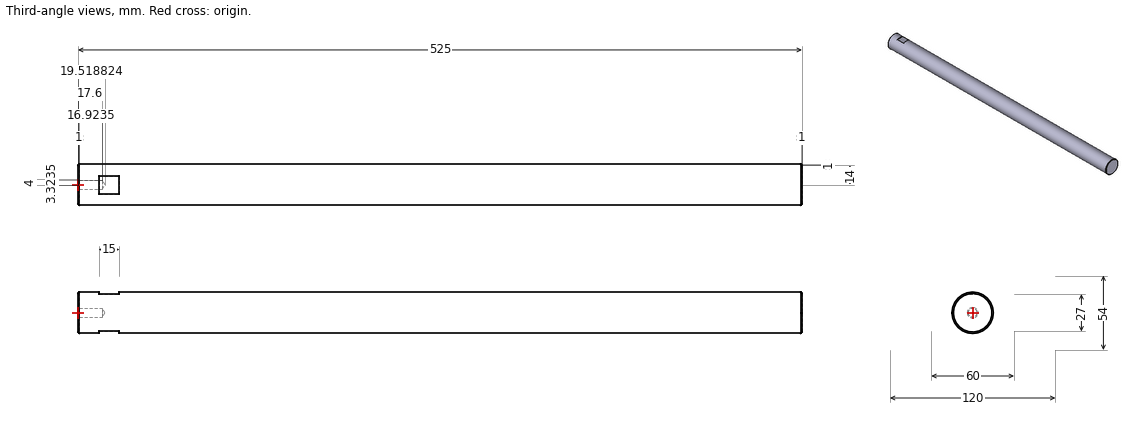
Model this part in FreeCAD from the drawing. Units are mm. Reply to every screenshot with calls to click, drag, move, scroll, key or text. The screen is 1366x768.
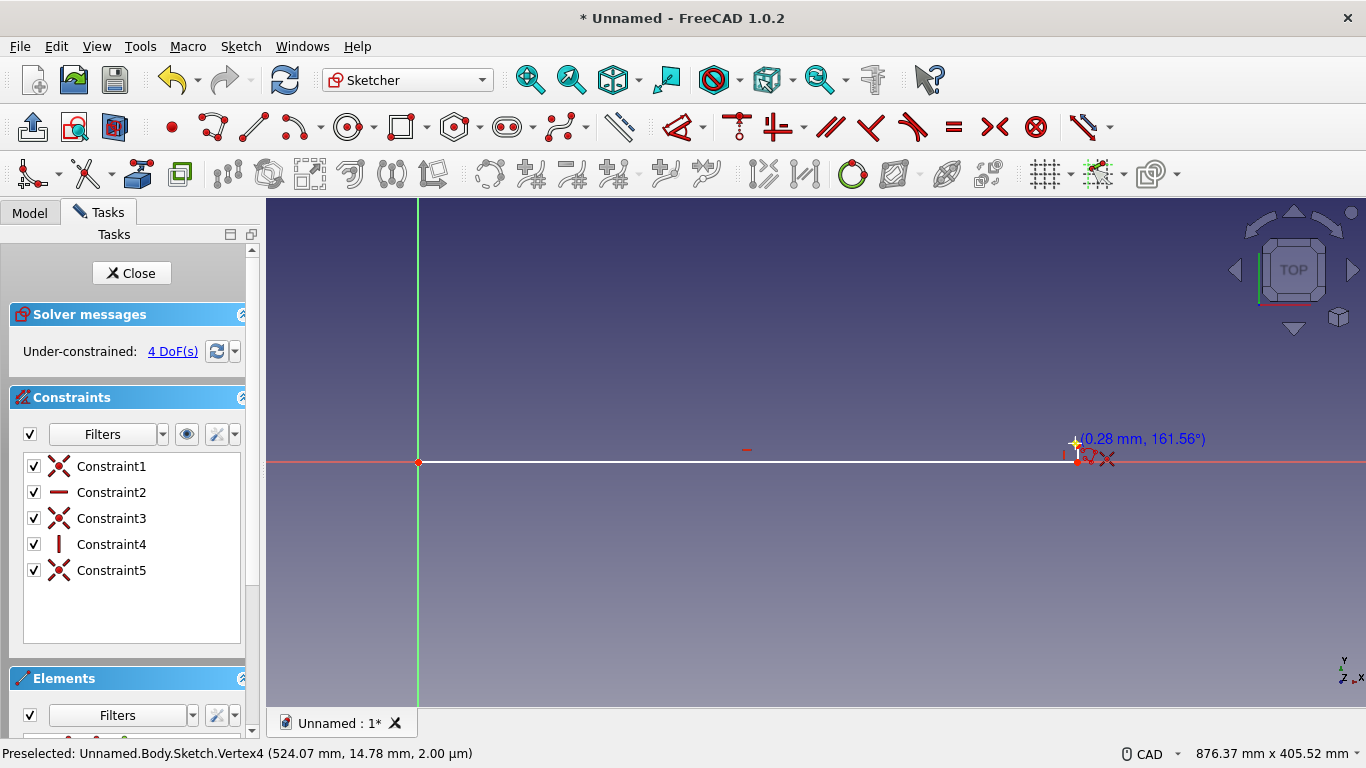
scroll(420, 443, up, 13)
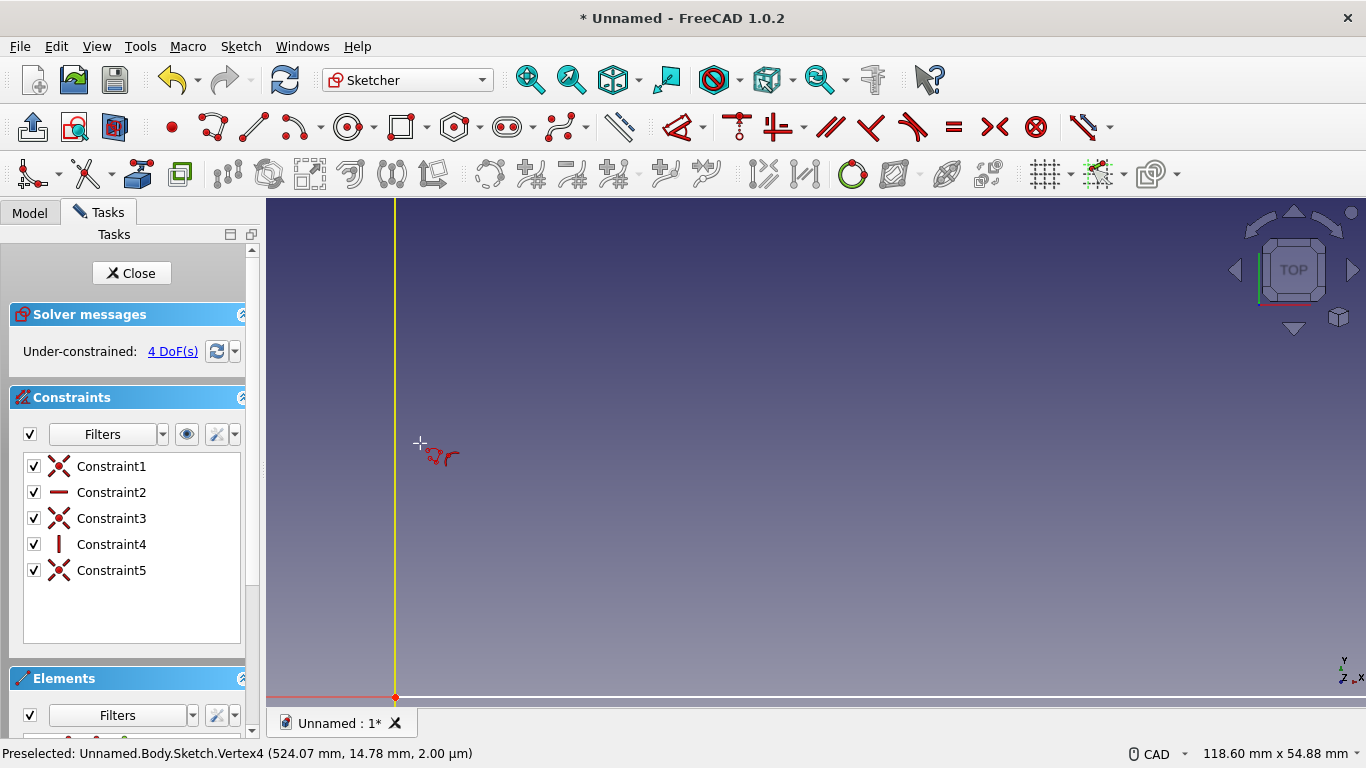
click(412, 444)
click(404, 460)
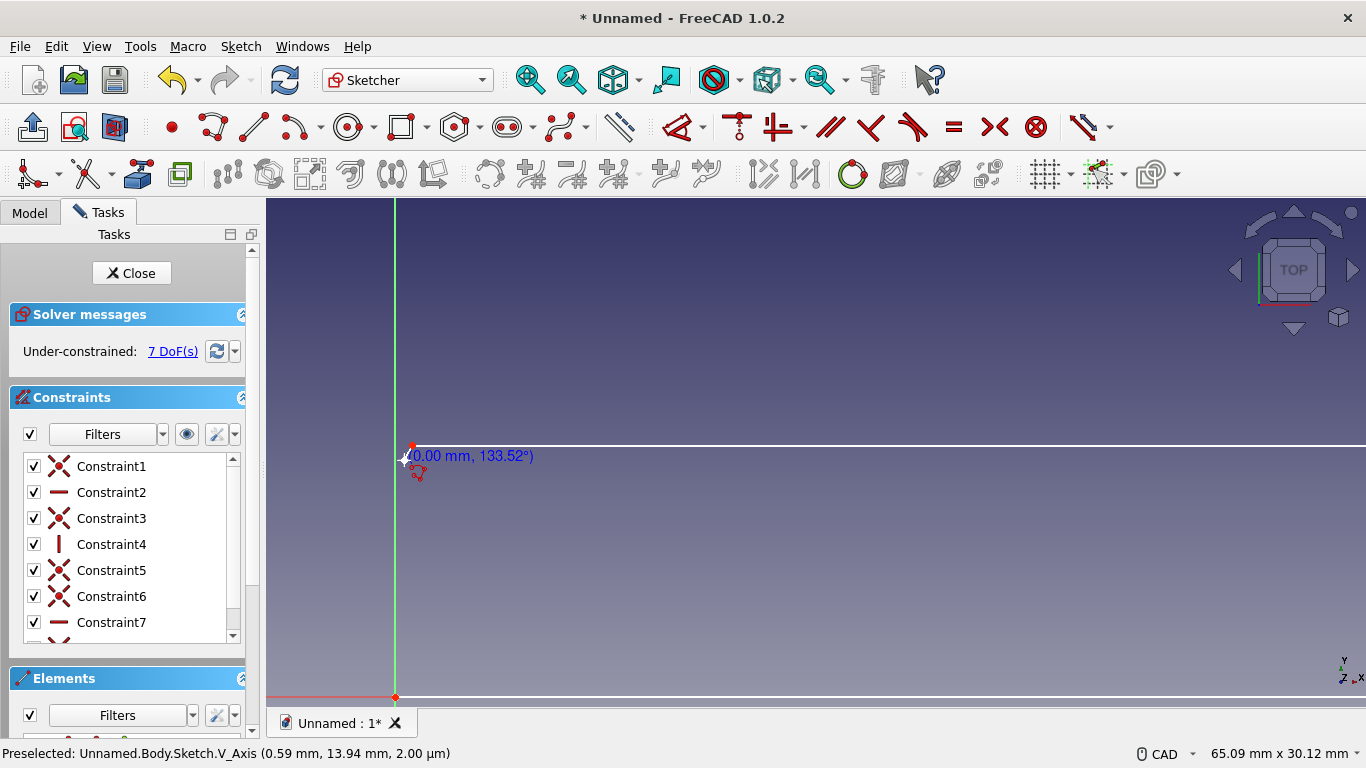
scroll(420, 443, down, 13)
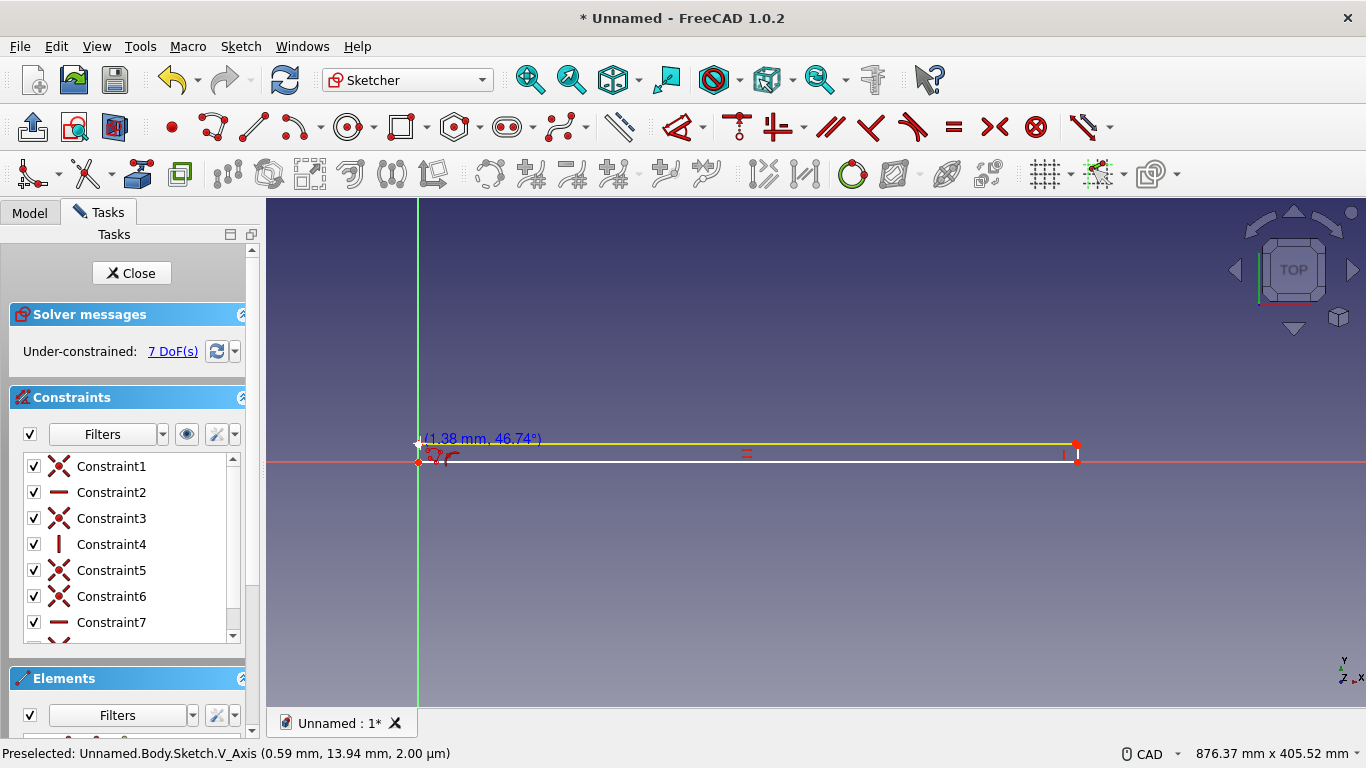
click(418, 462)
key(Escape)
key(Escape)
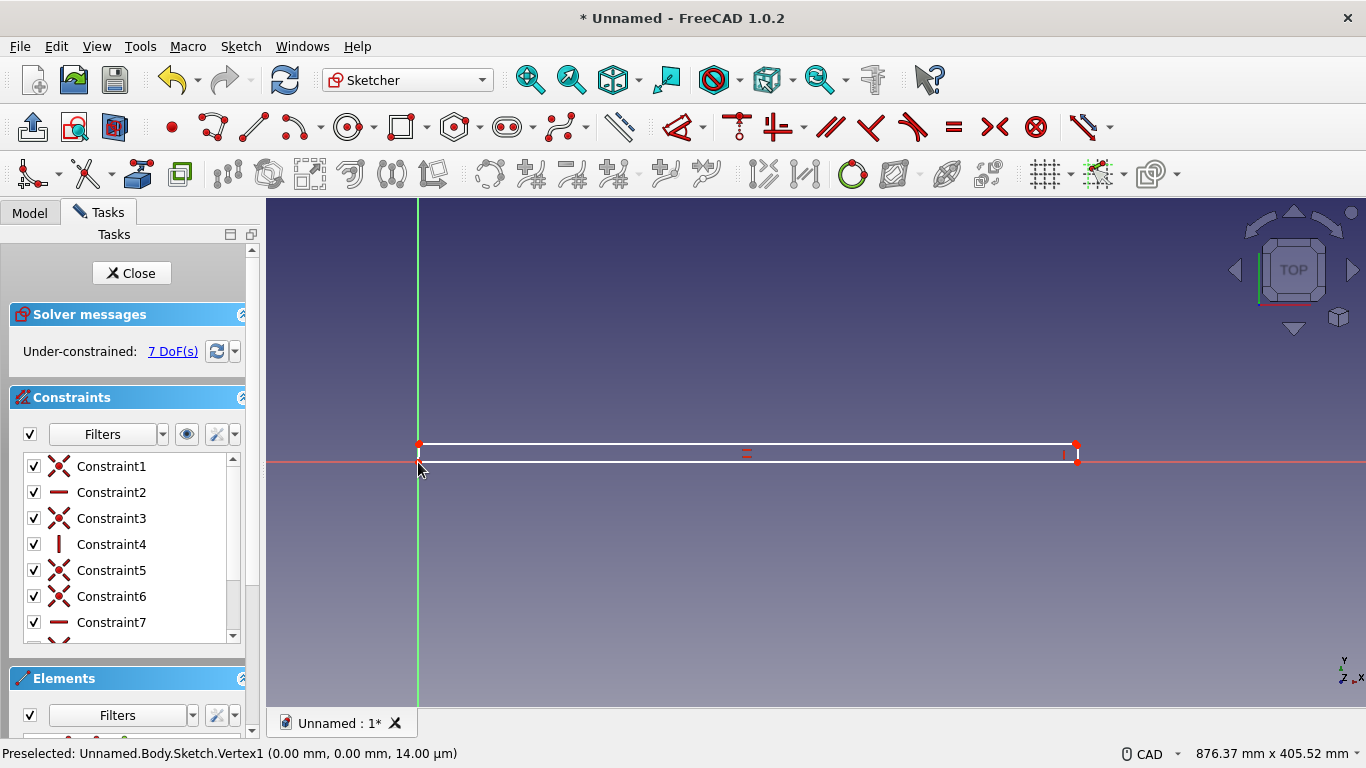
scroll(419, 454, up, 3)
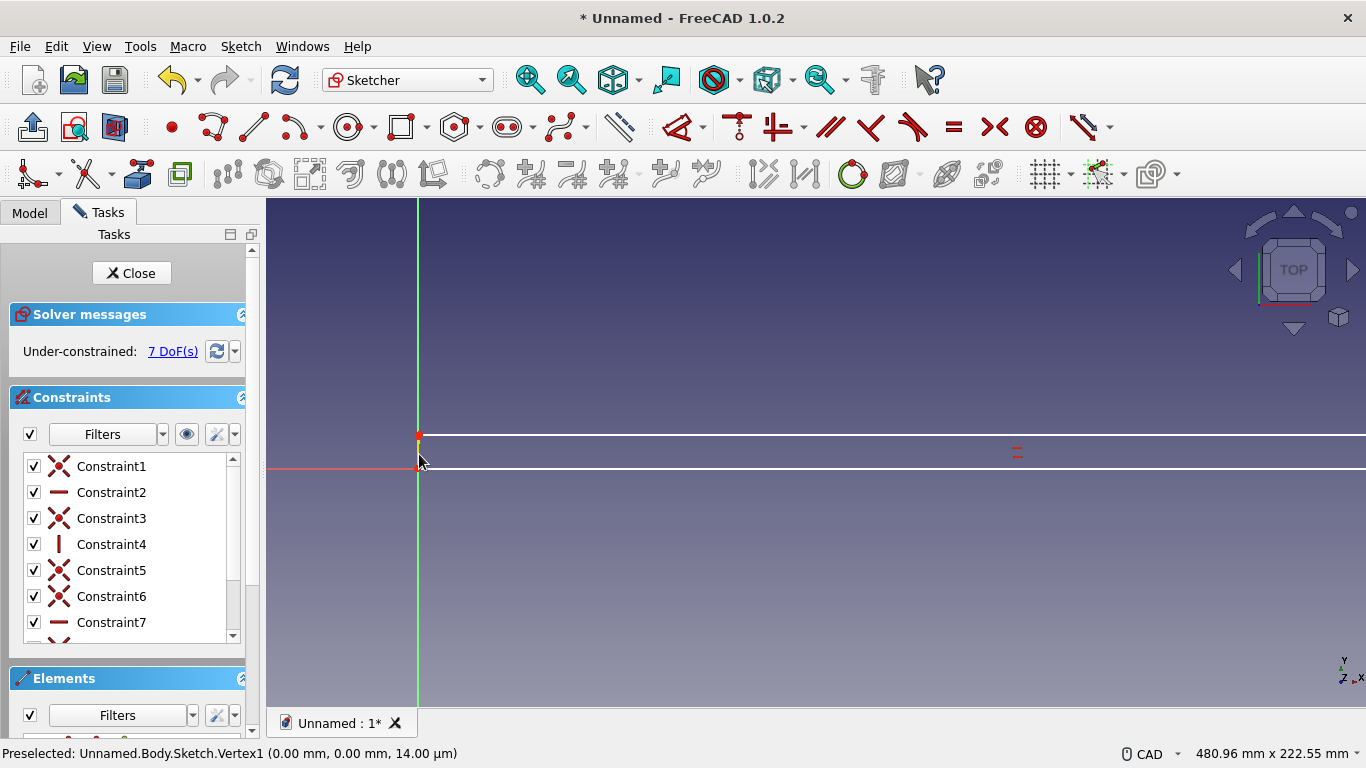
click(418, 453)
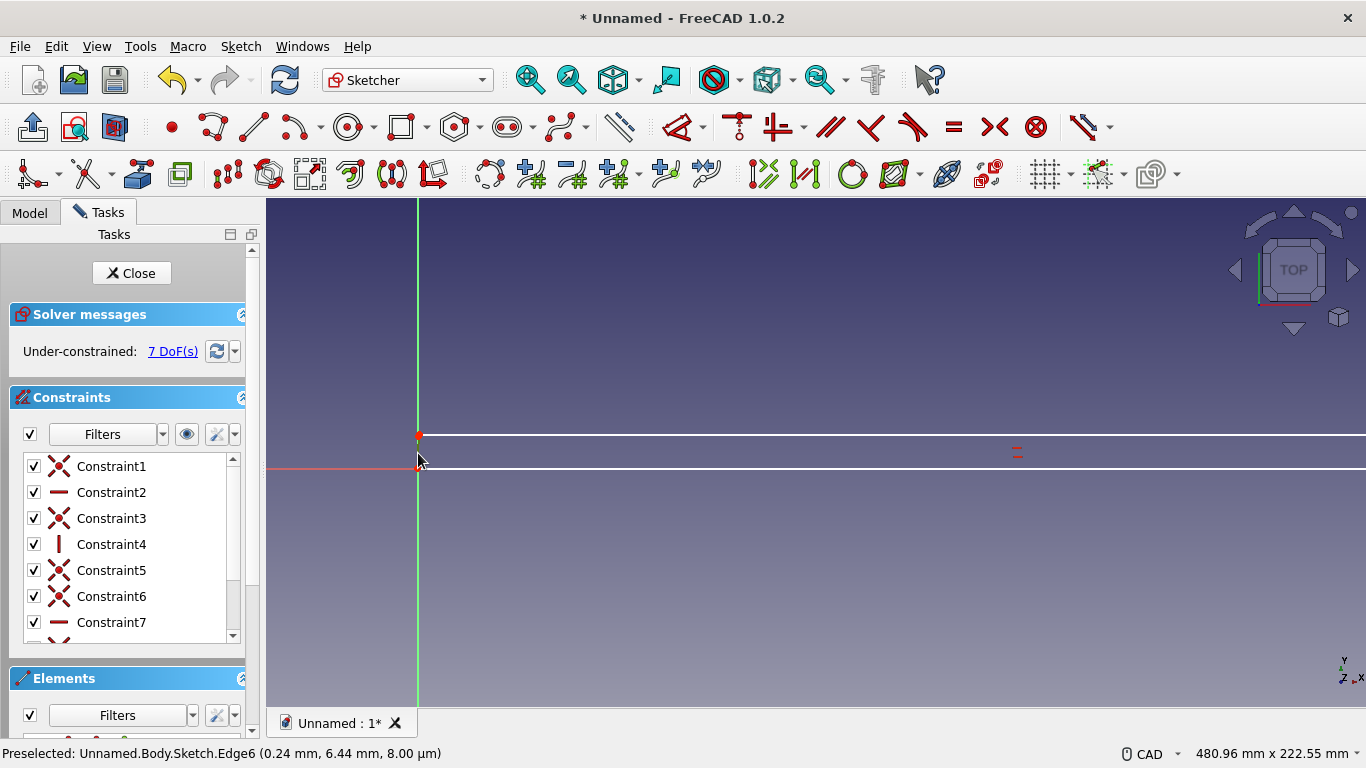
click(804, 128)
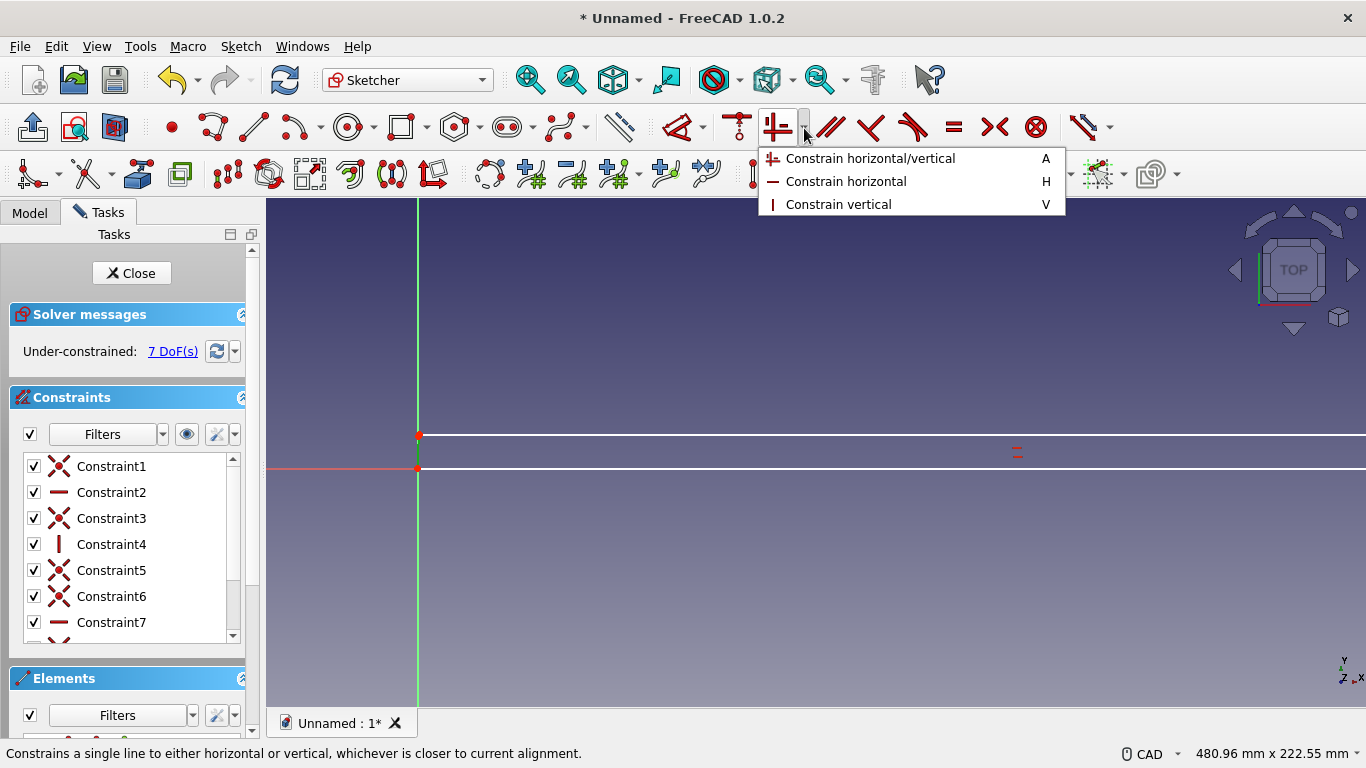
click(912, 204)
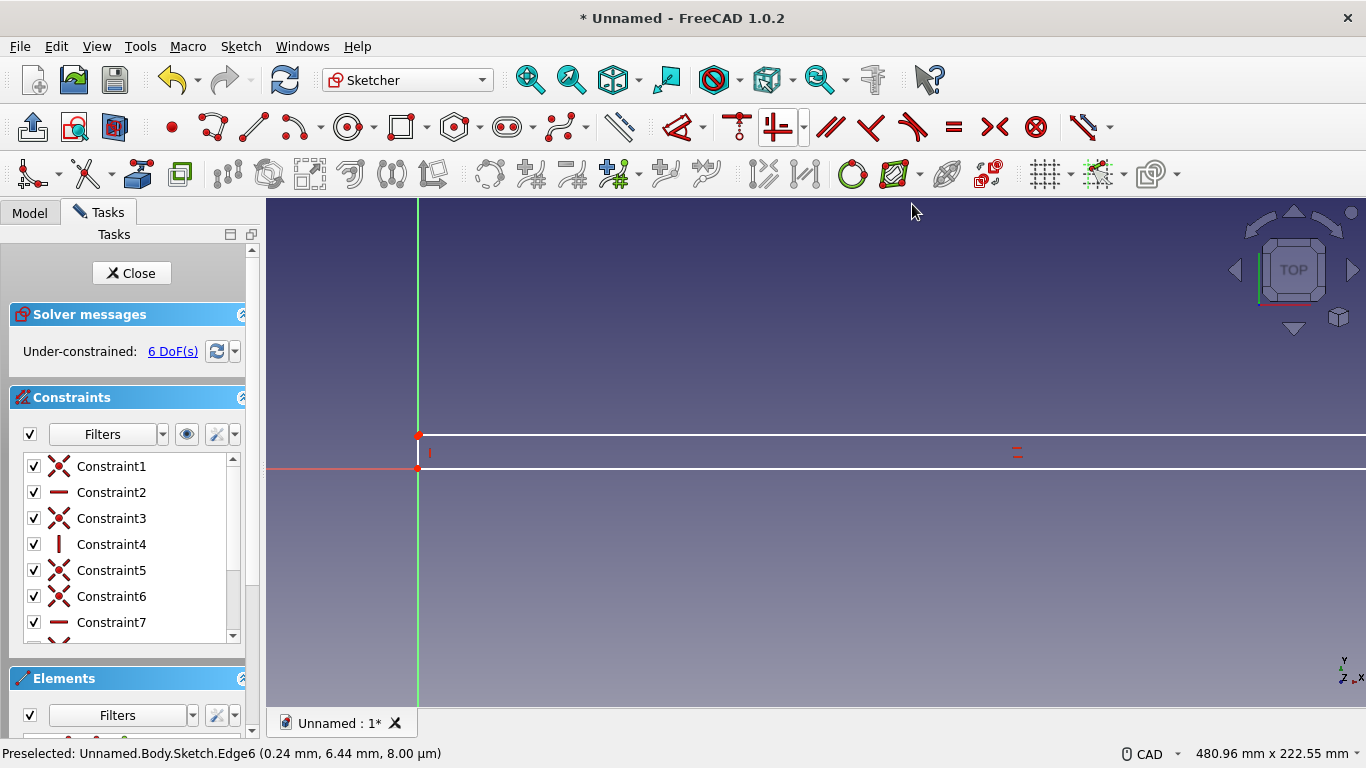
click(676, 128)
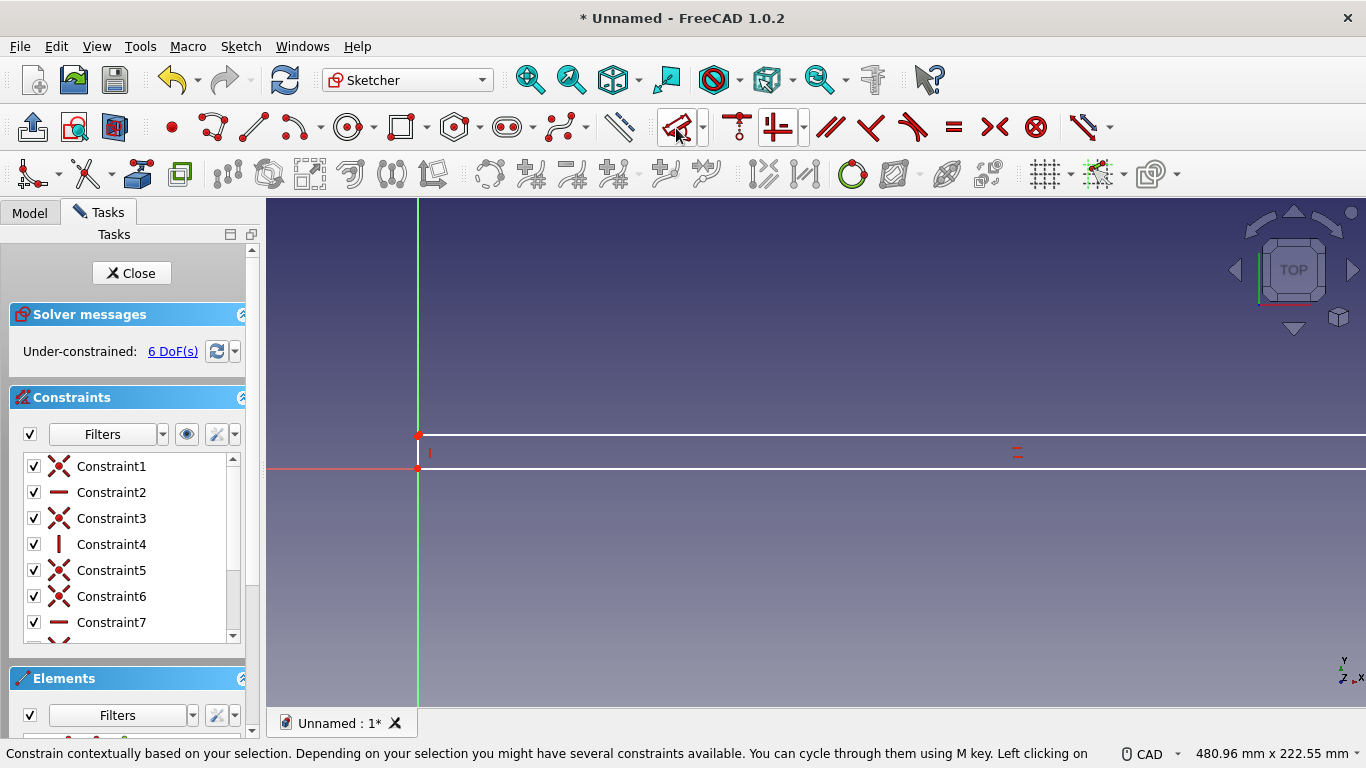
scroll(419, 454, down, 3)